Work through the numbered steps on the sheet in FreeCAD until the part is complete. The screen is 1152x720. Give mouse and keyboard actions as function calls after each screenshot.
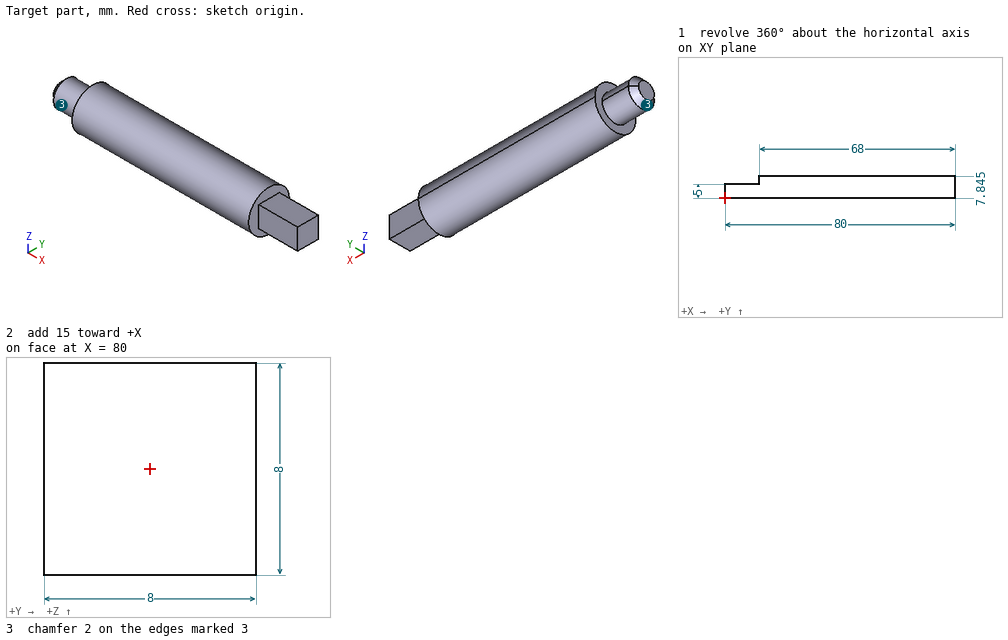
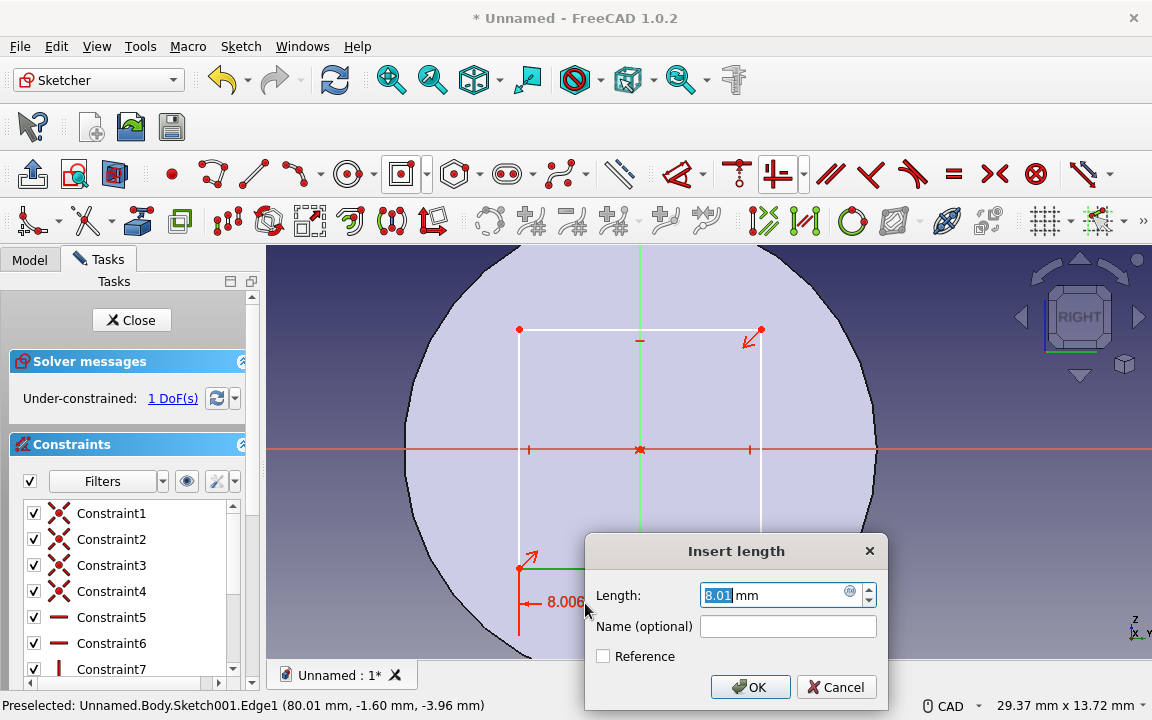
text(8)
key(Return)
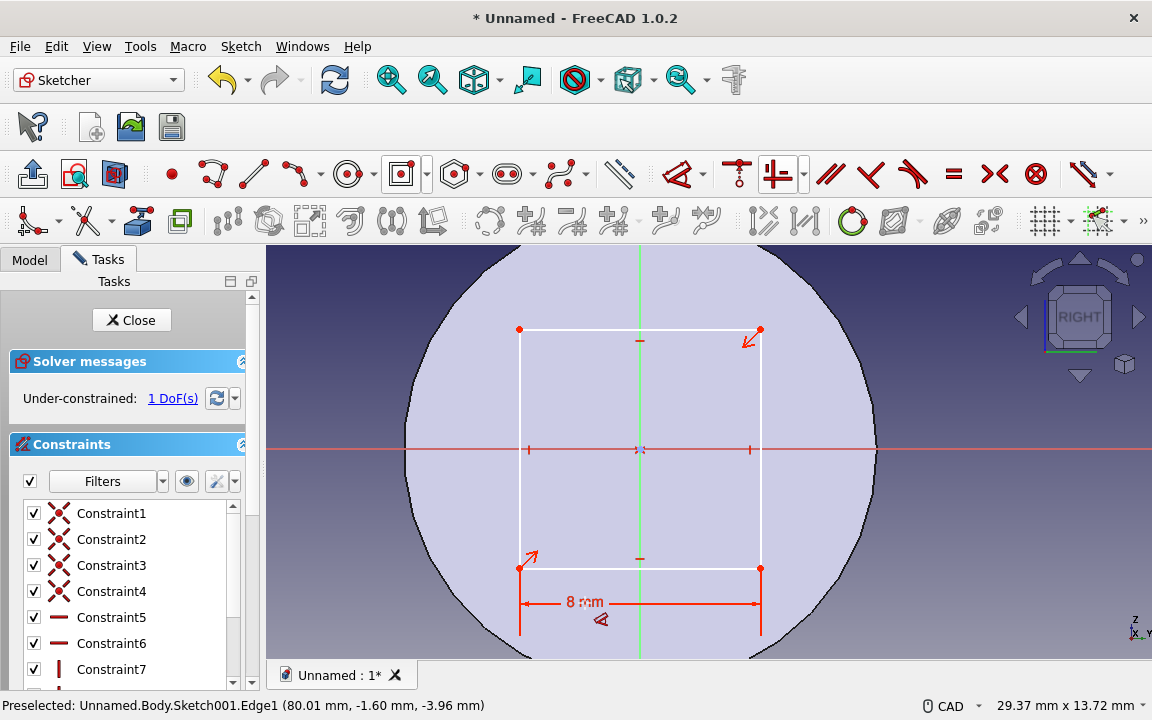
click(761, 497)
click(795, 395)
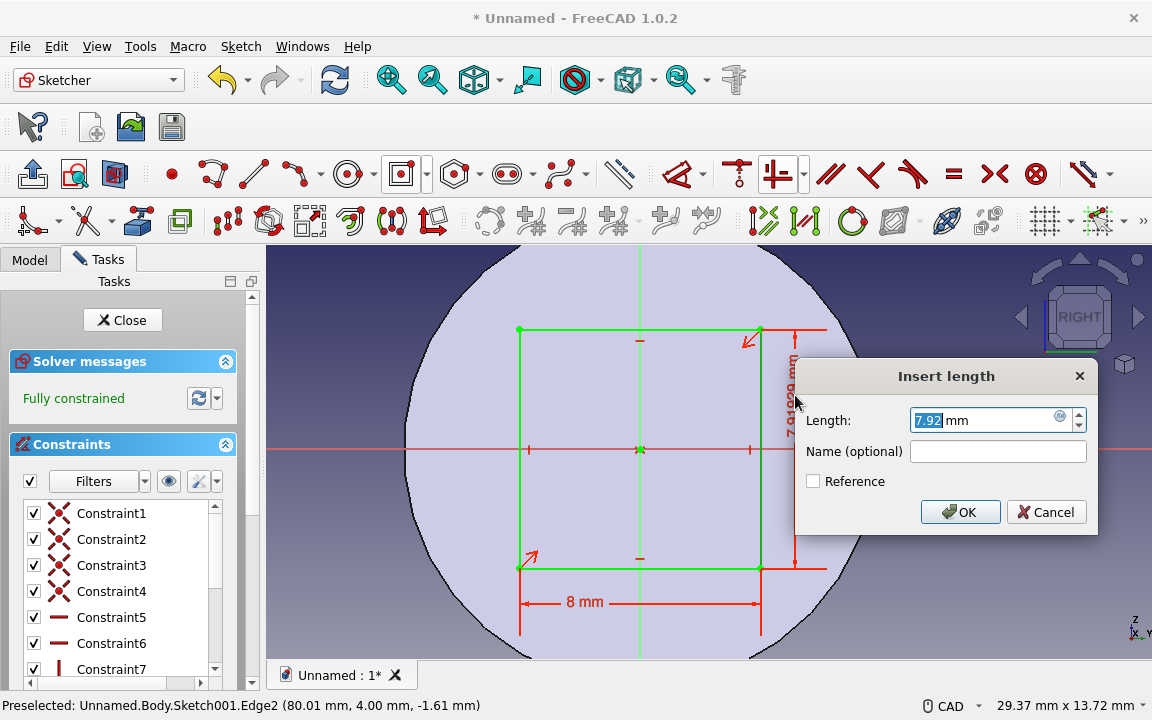
text(8)
key(Return)
key(Escape)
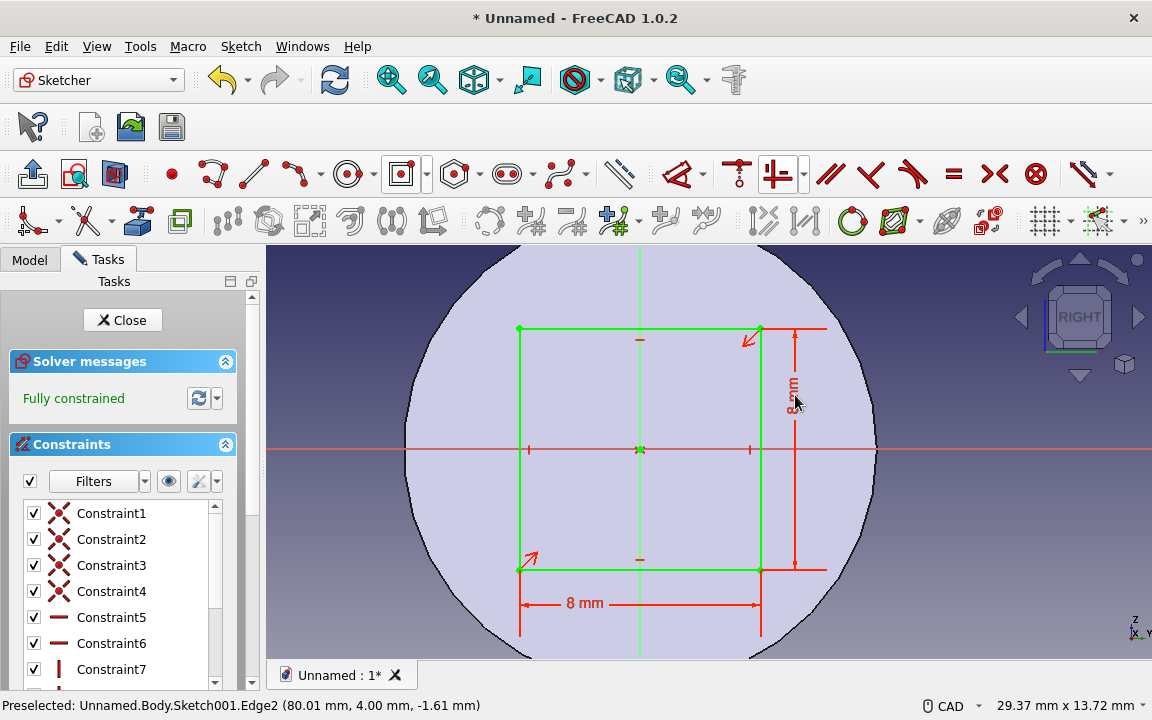
click(123, 320)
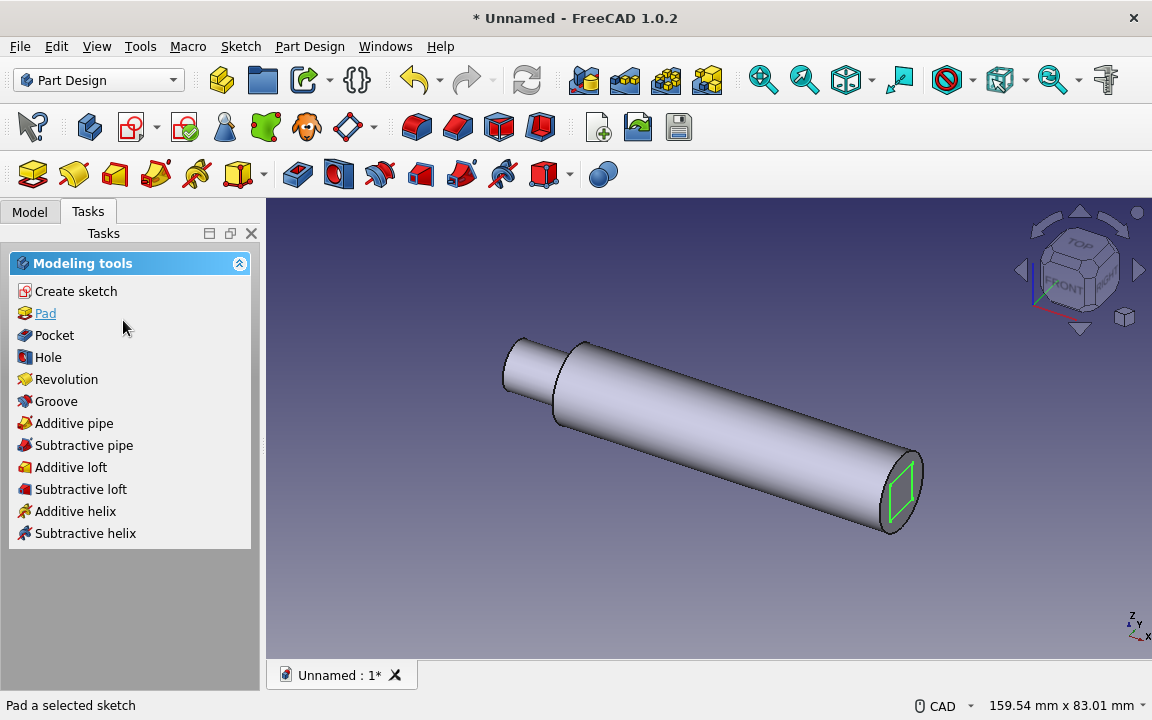
click(33, 174)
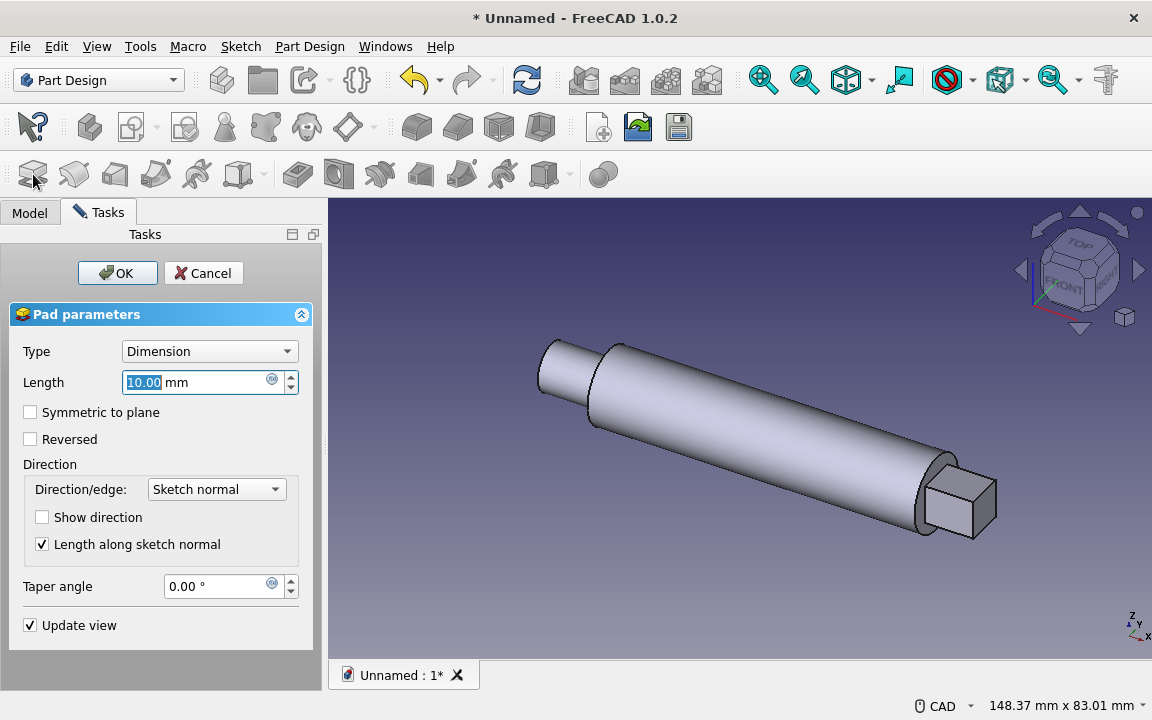
text(15)
key(Tab)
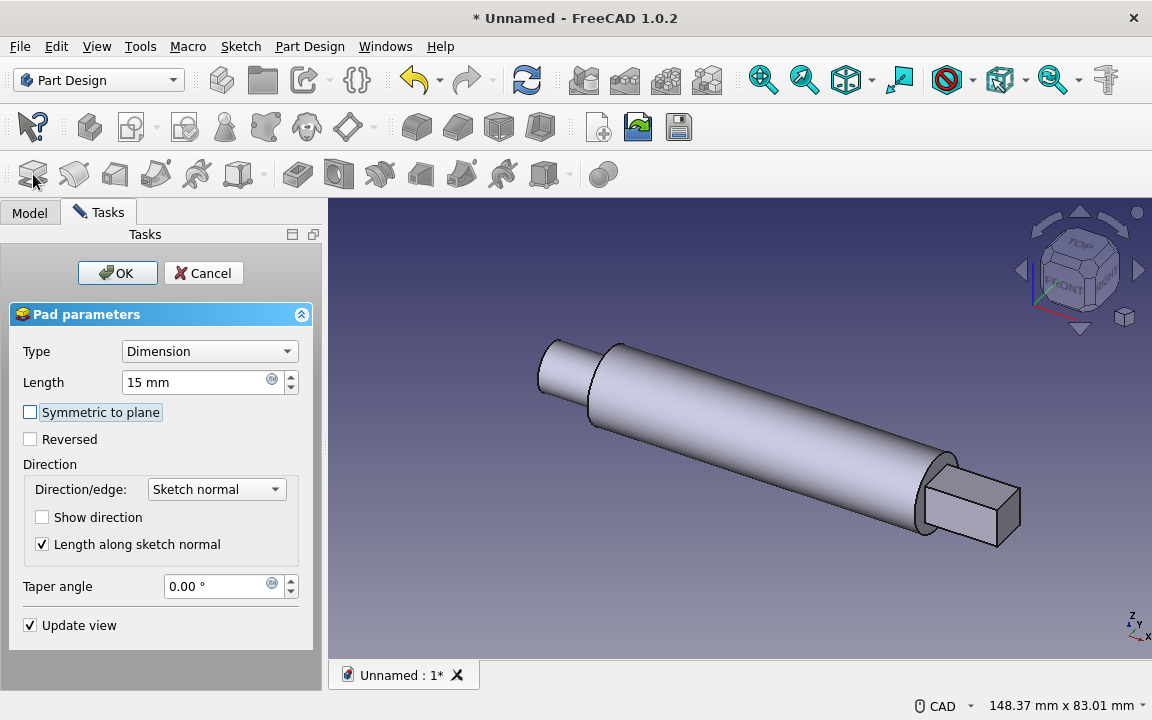
click(118, 273)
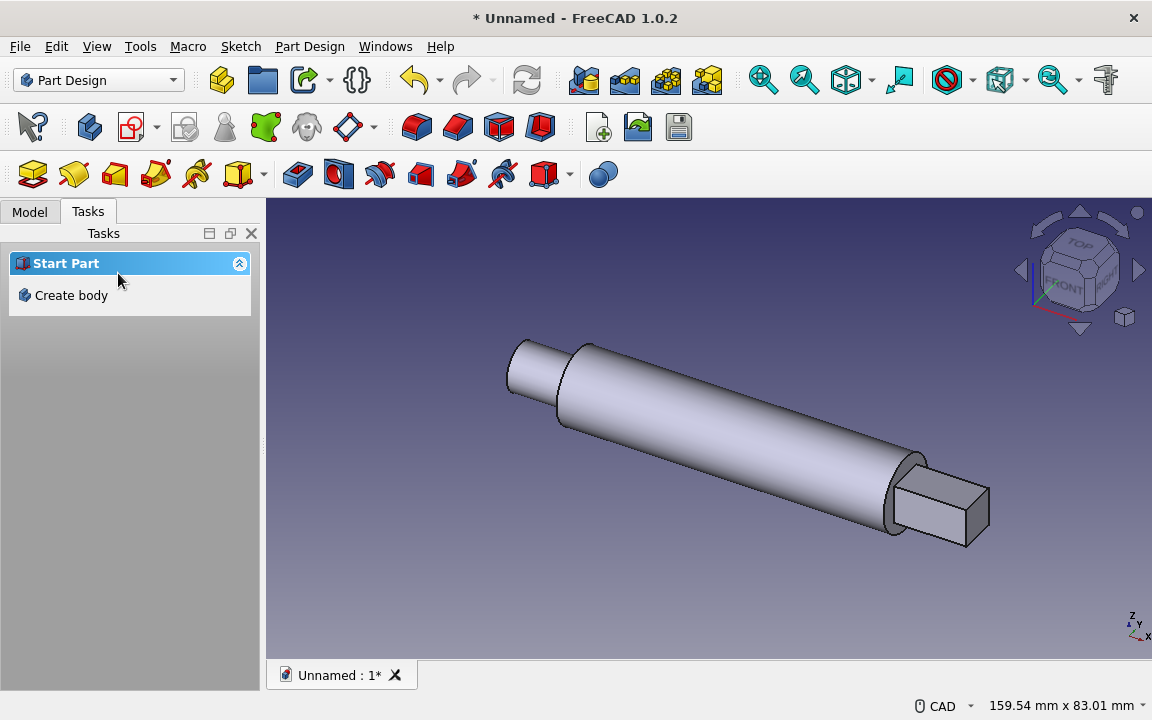
click(509, 390)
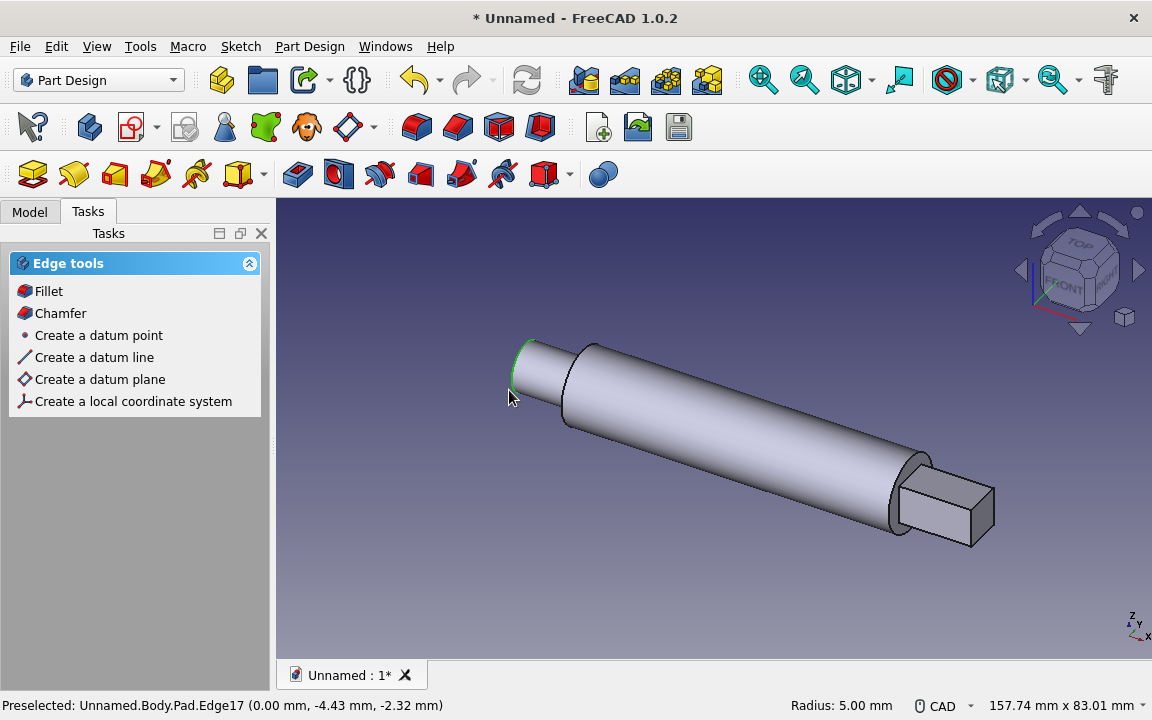
click(458, 128)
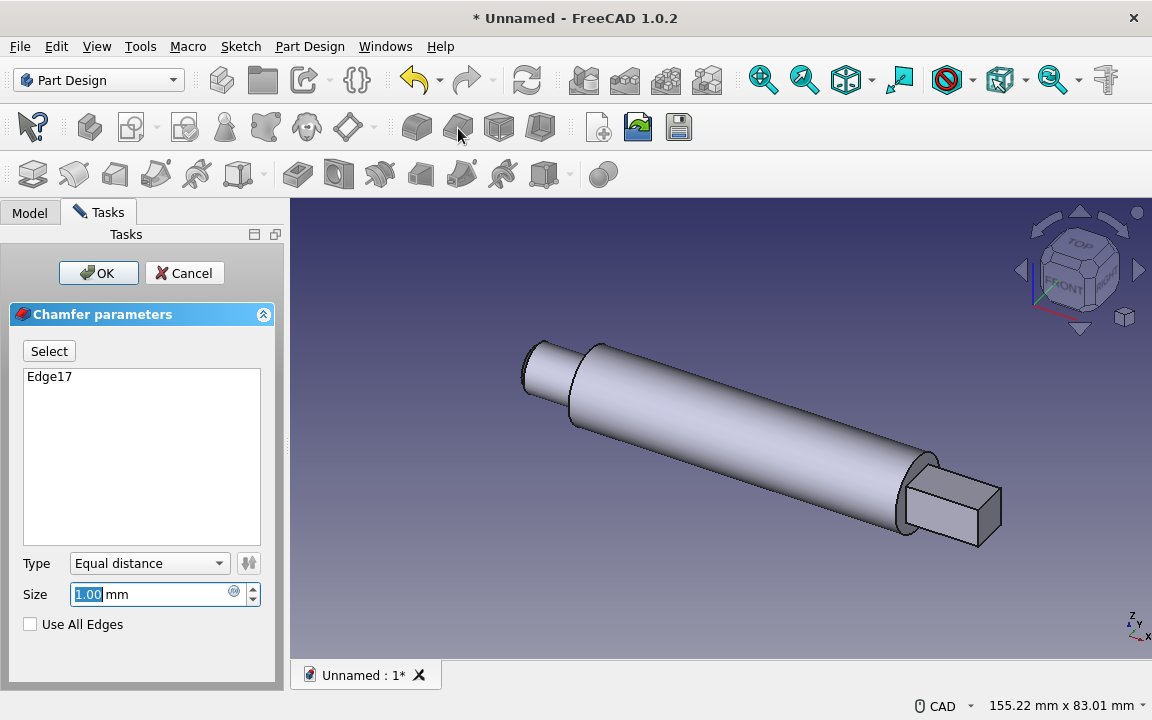
text(2)
key(Tab)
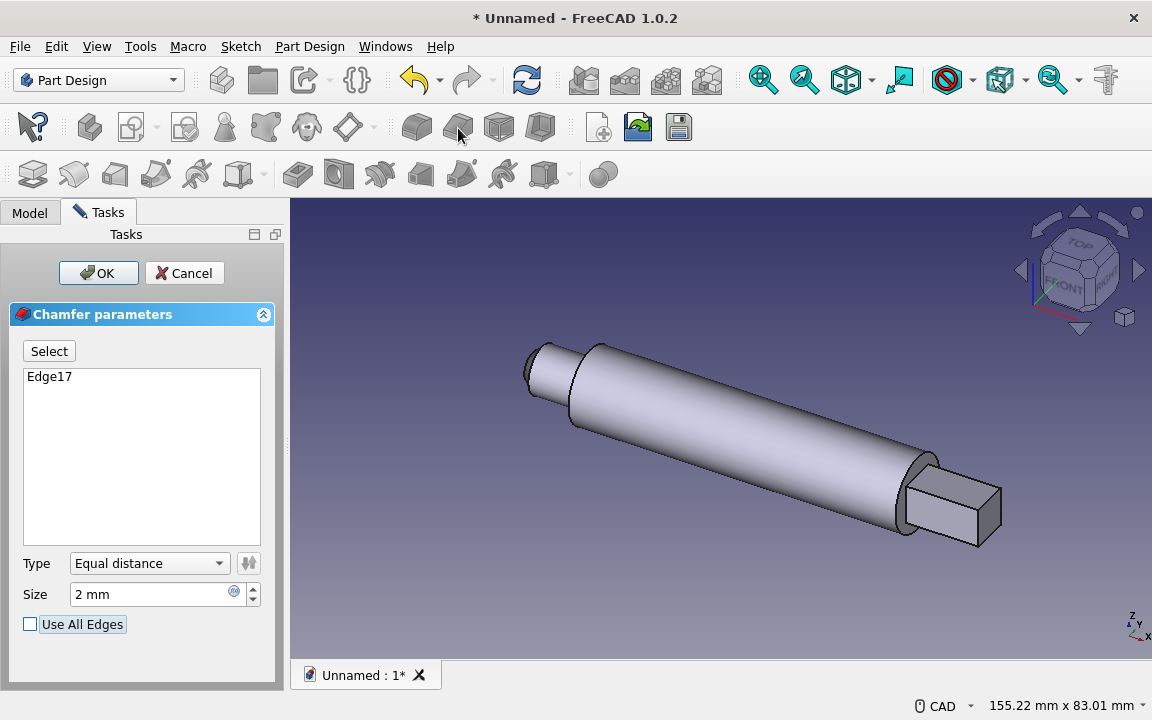
click(99, 273)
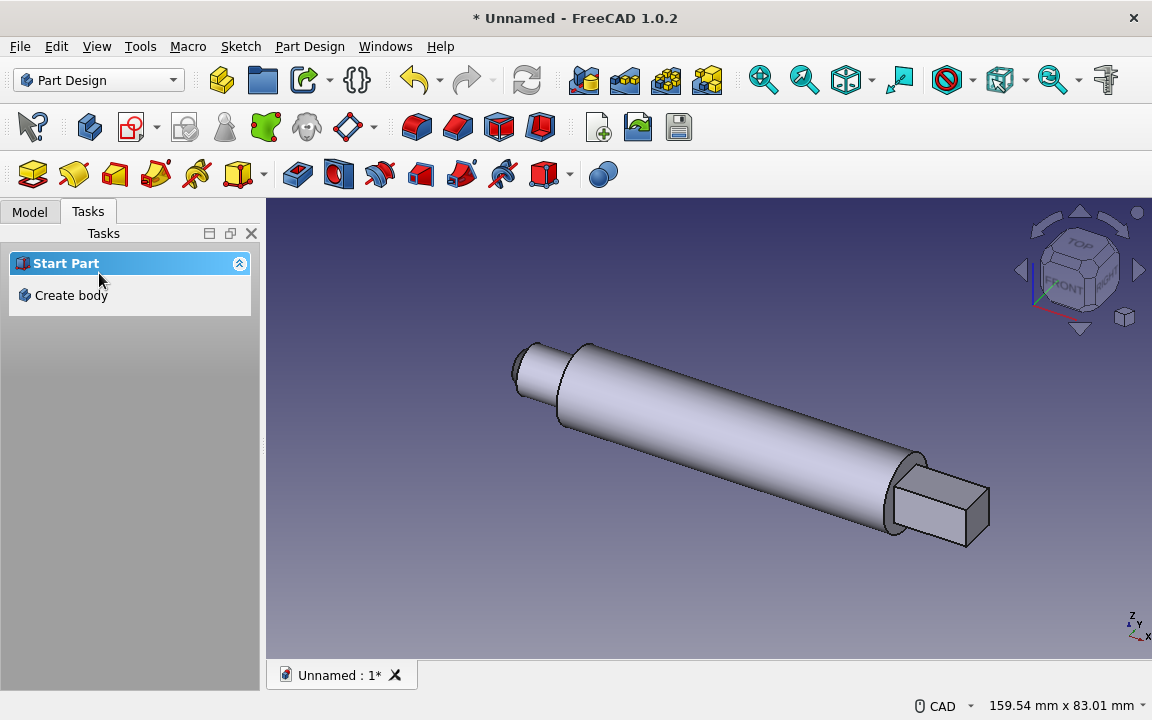
key(0)